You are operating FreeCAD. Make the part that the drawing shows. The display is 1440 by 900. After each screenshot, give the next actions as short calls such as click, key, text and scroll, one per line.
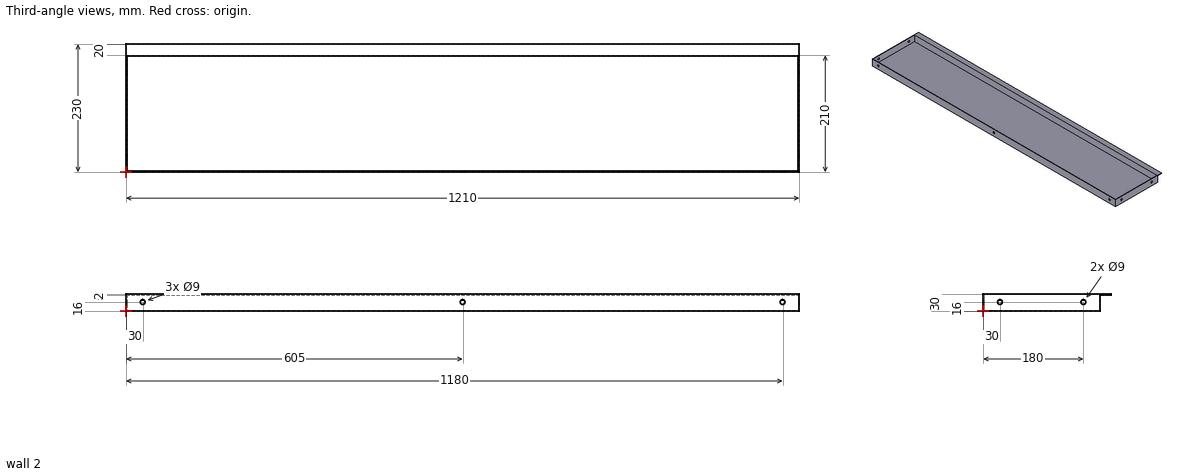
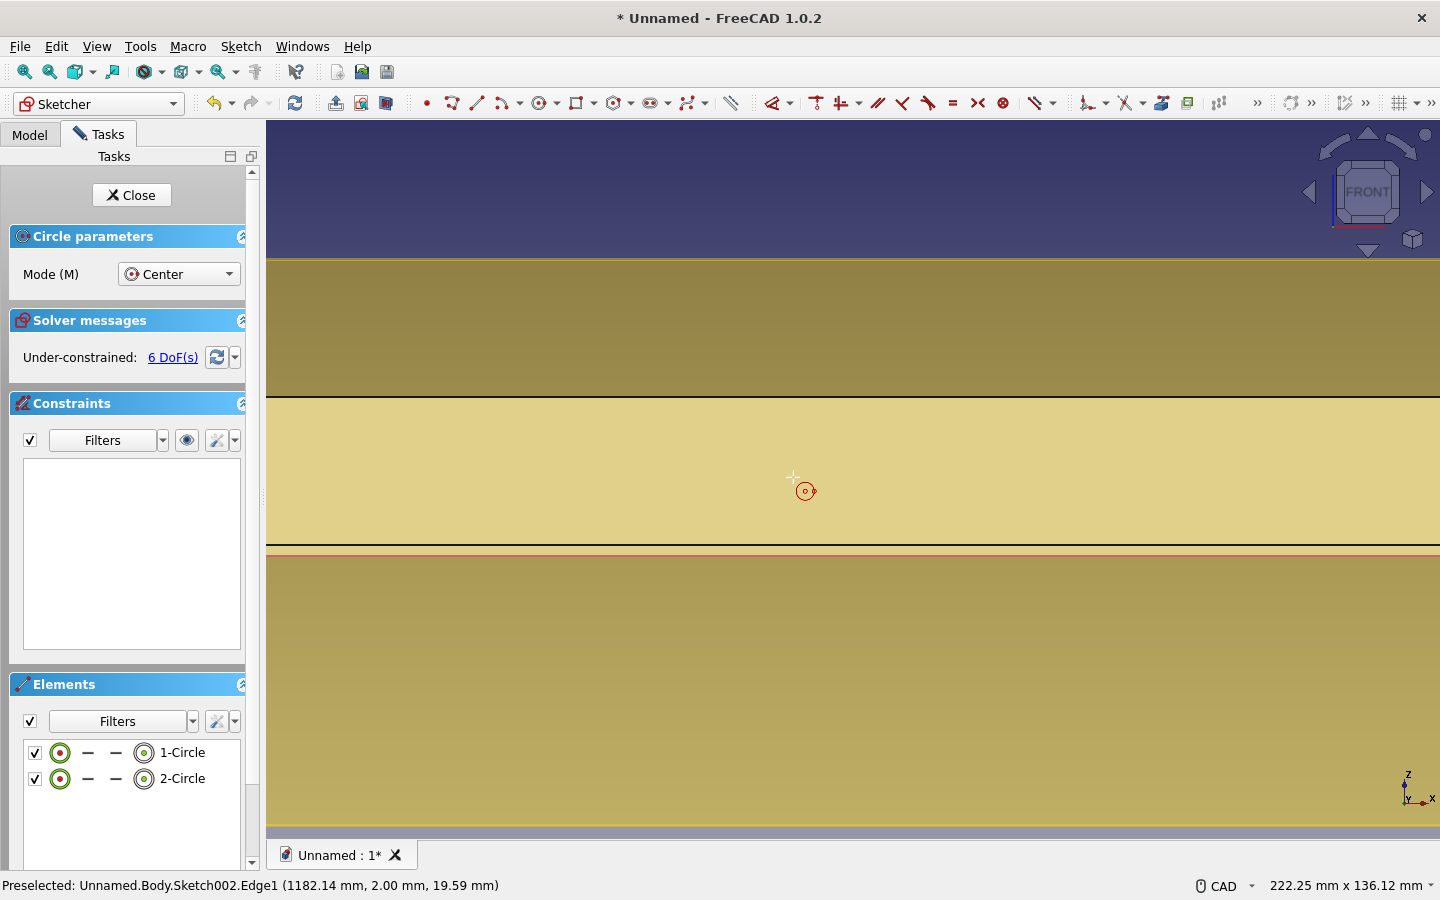
scroll(793, 477, down, 11)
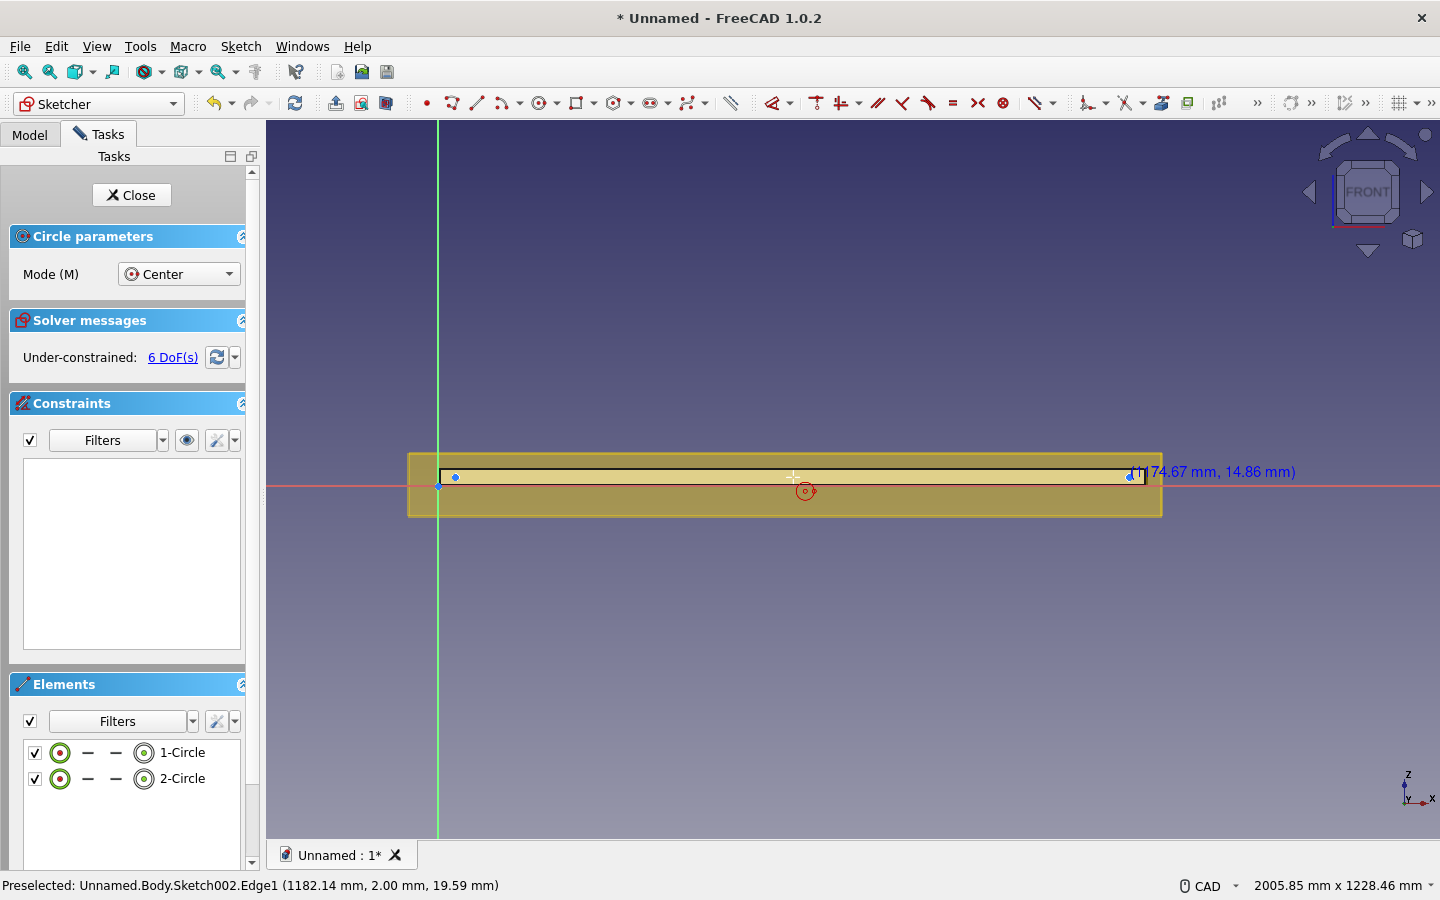
scroll(793, 477, up, 3)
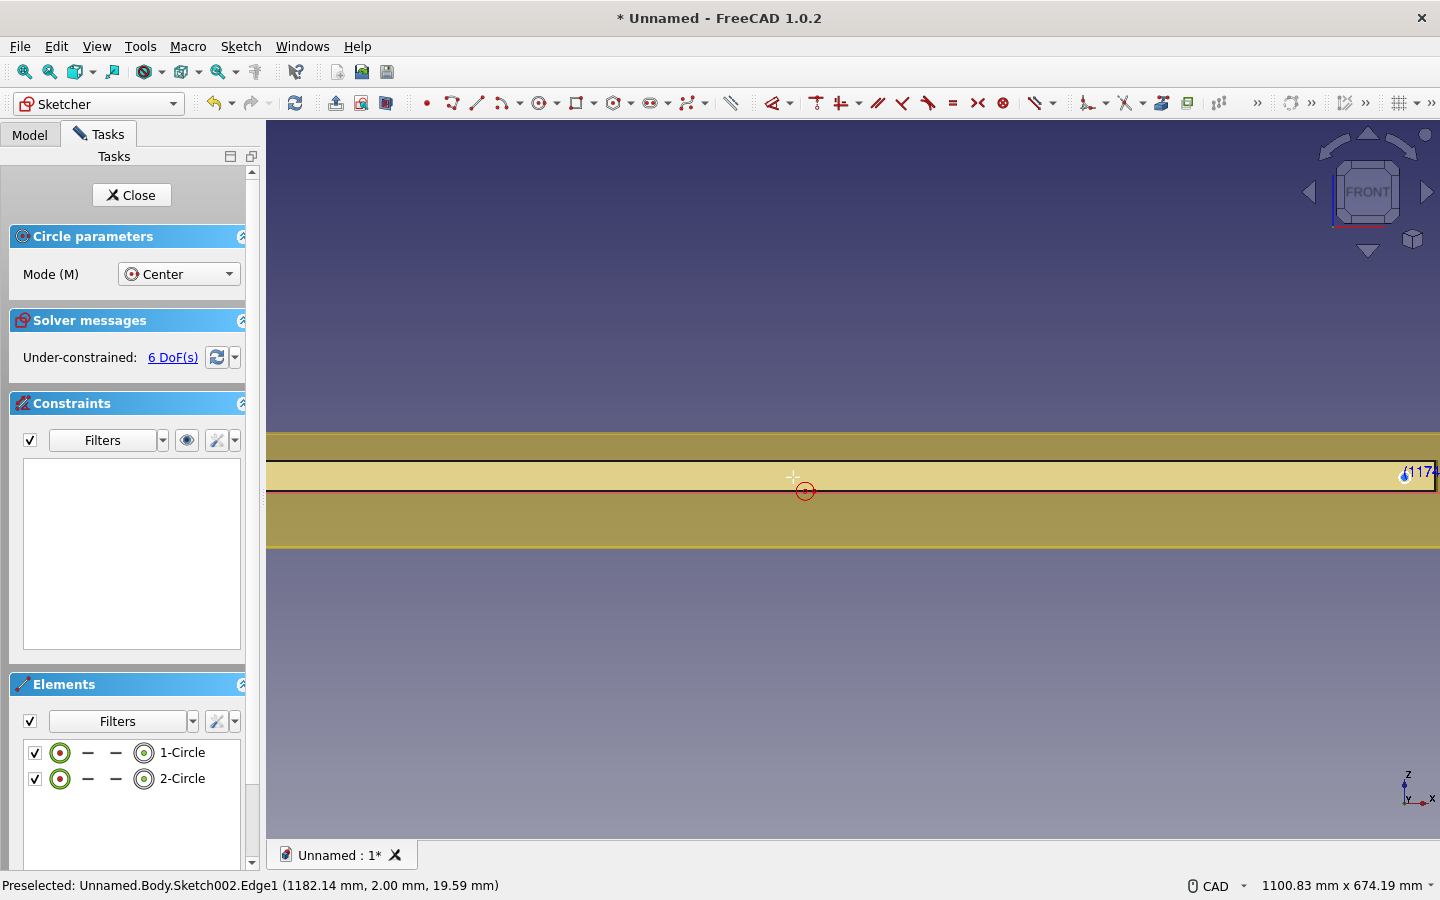
click(792, 476)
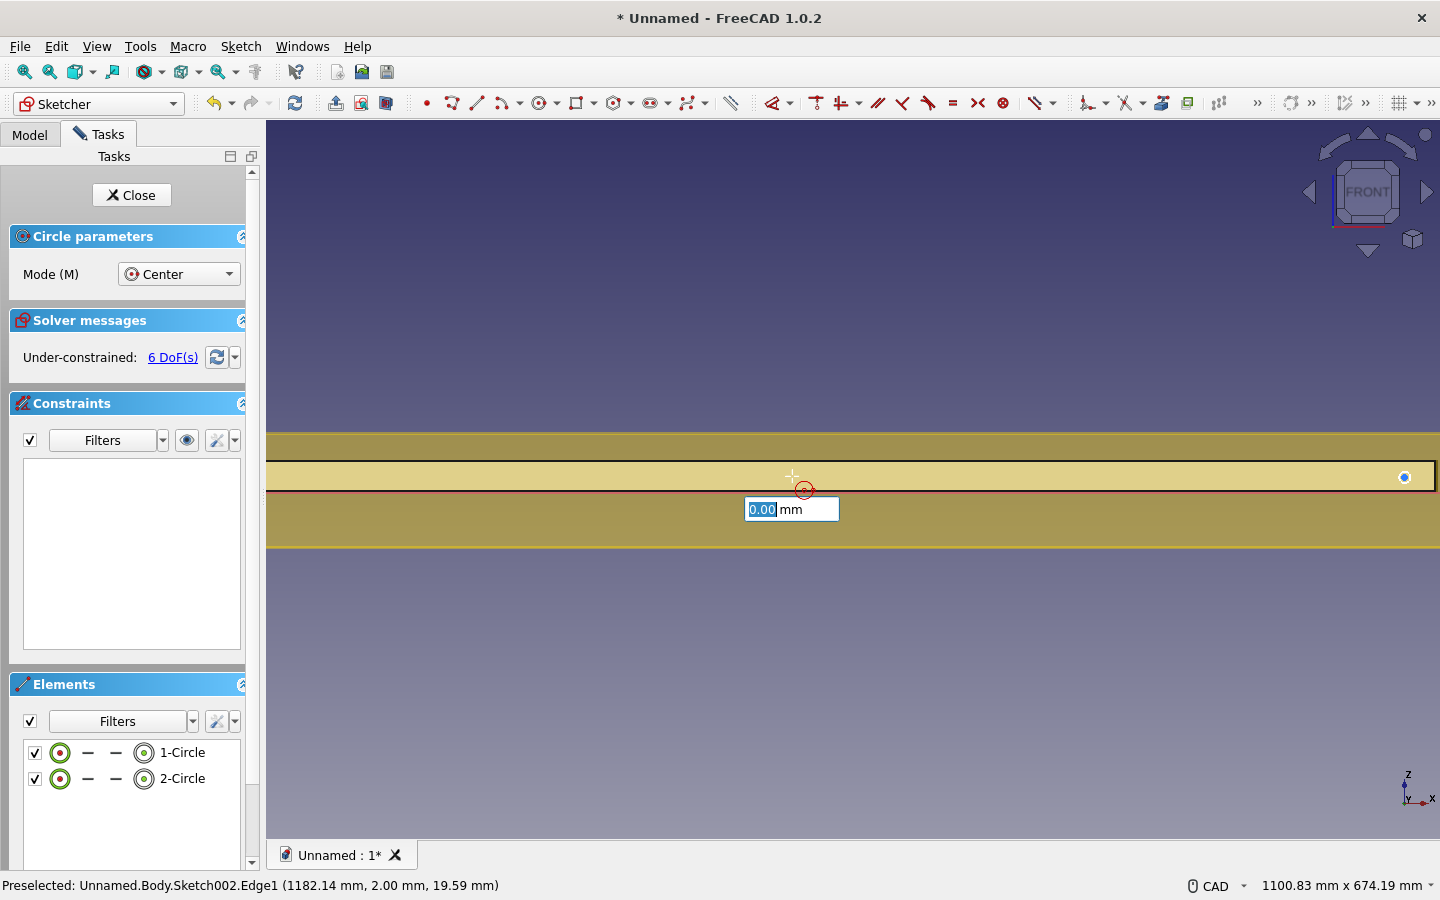
scroll(795, 473, up, 6)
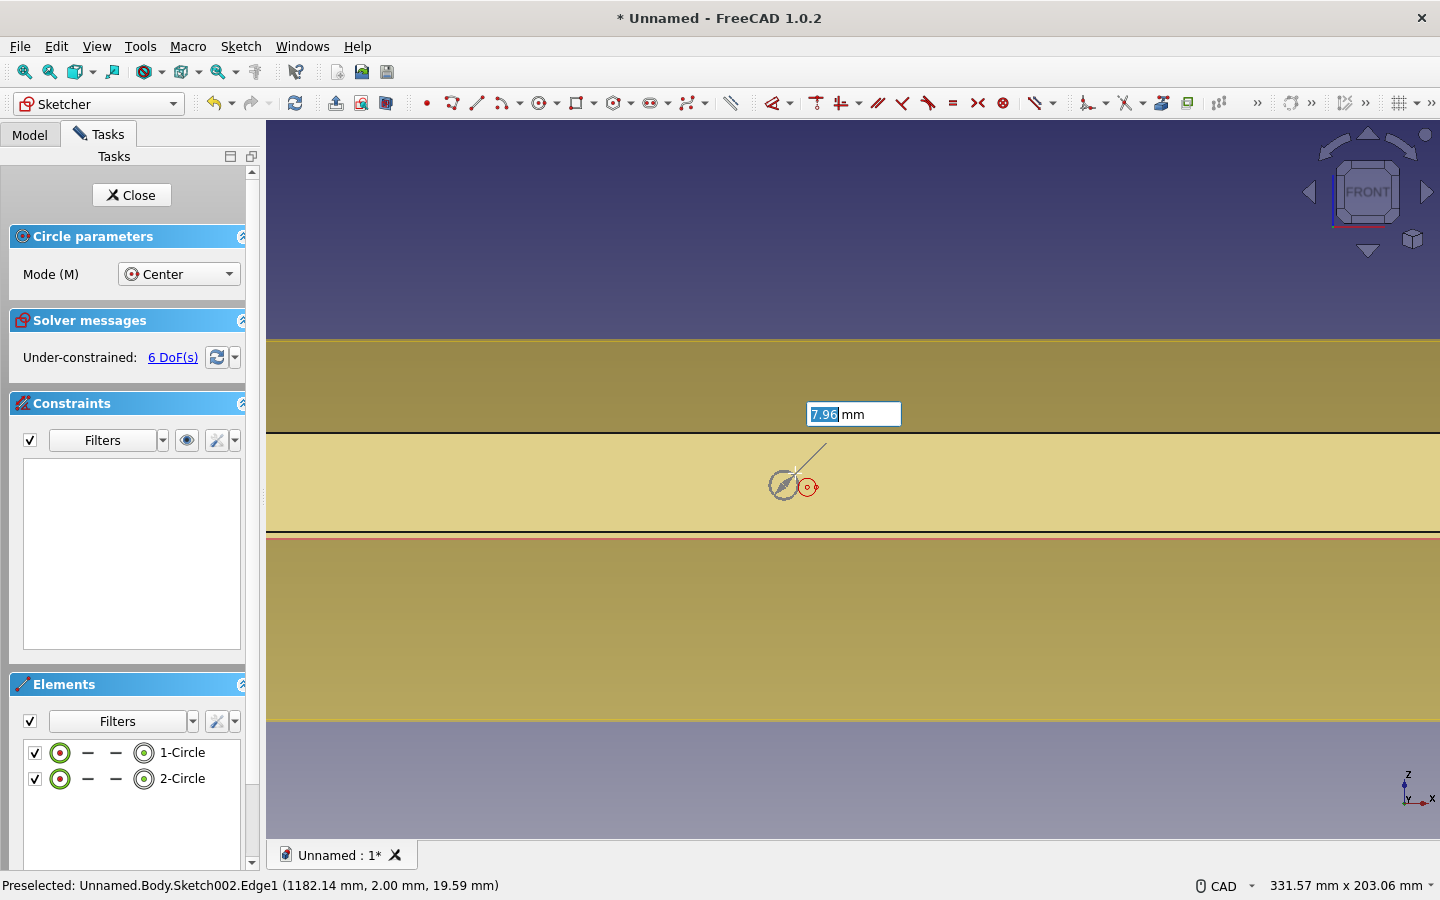
click(794, 471)
key(Escape)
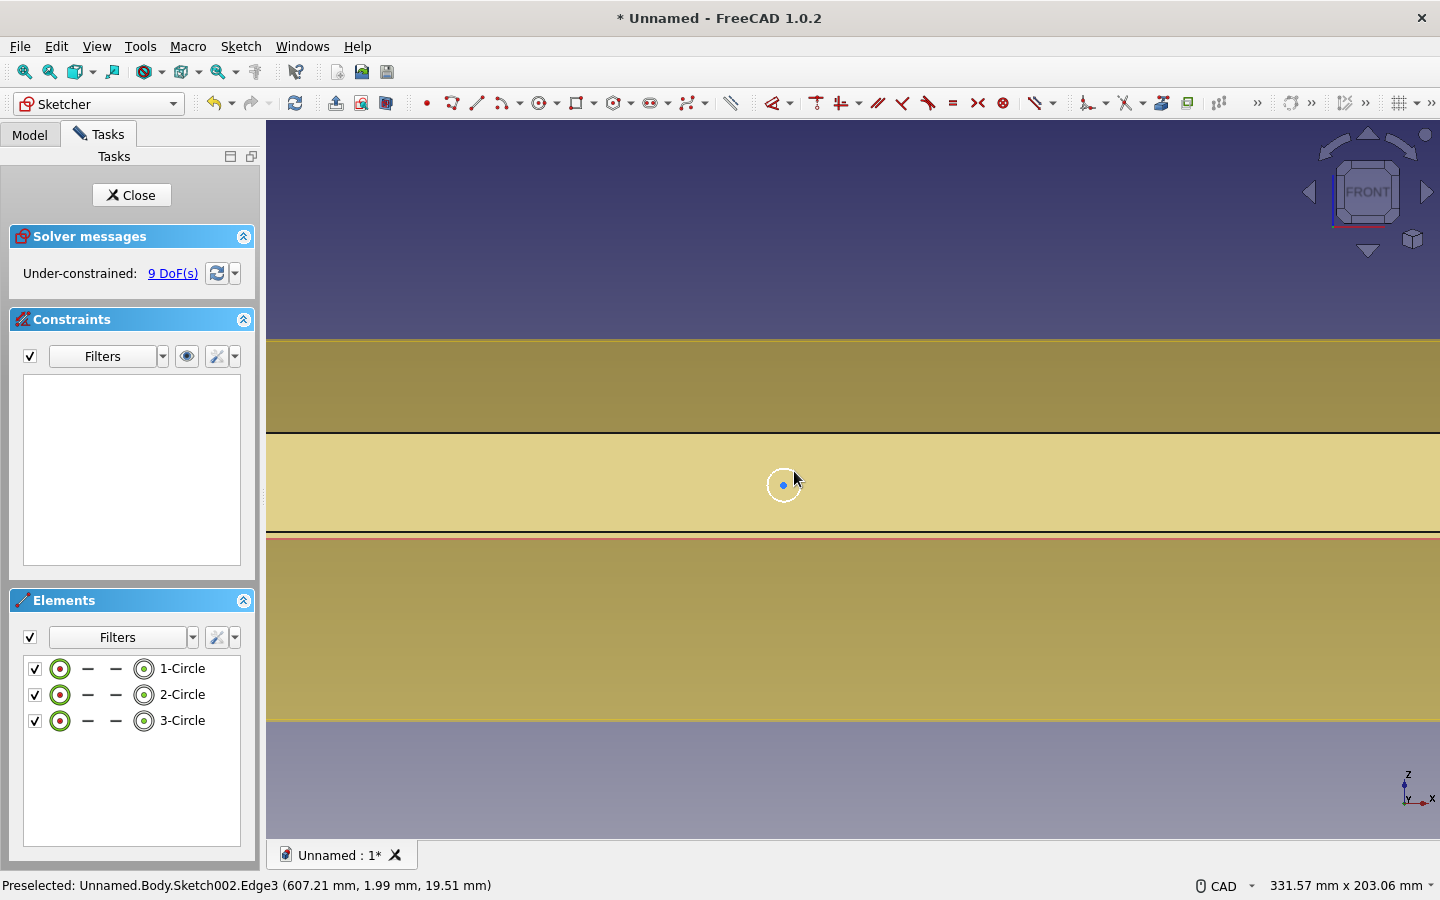
scroll(794, 475, down, 9)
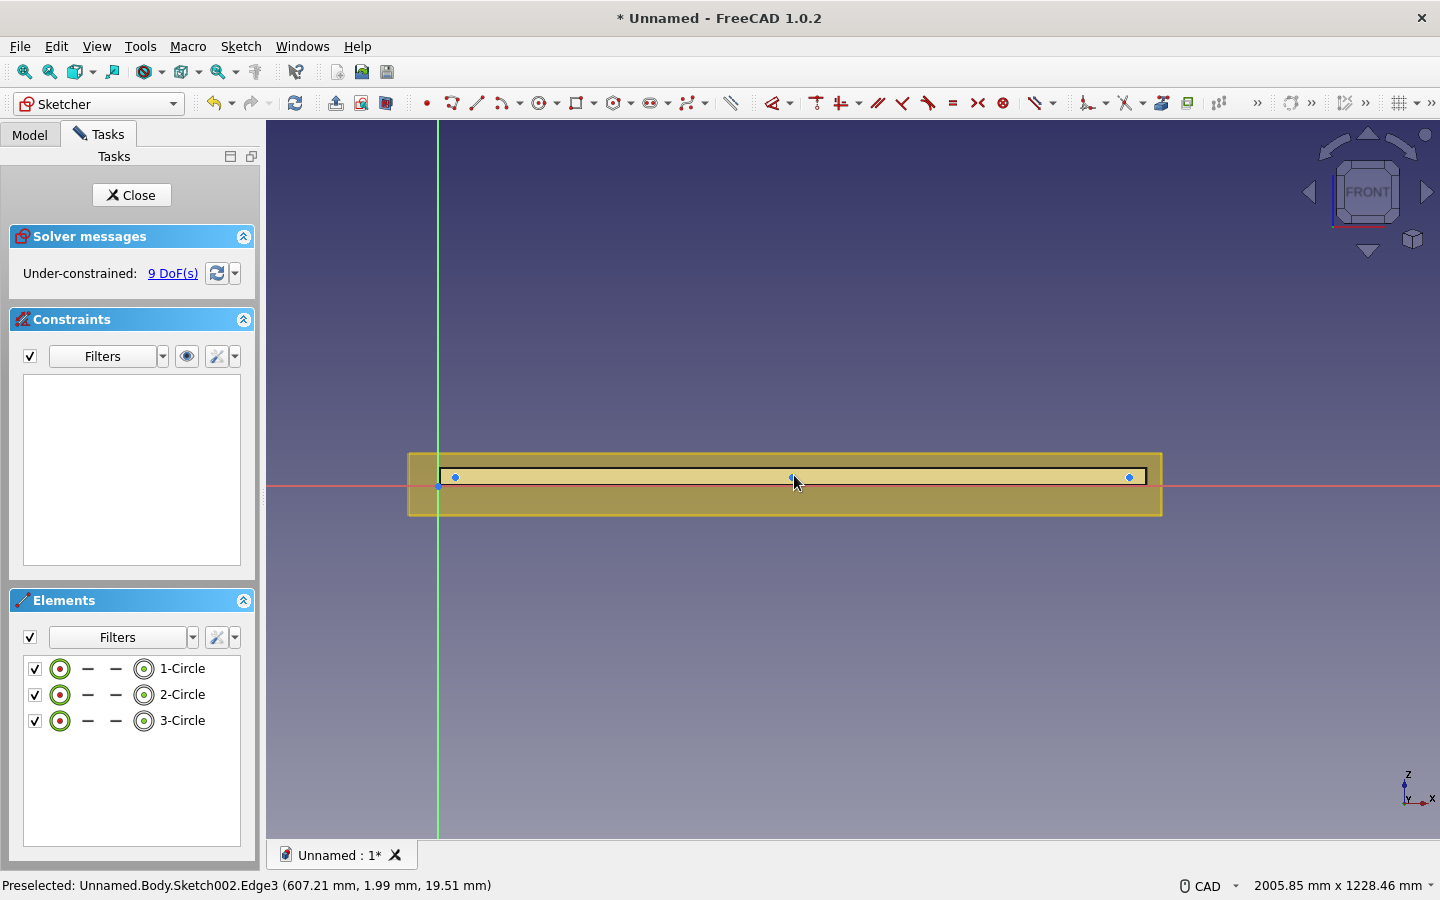
scroll(458, 475, up, 8)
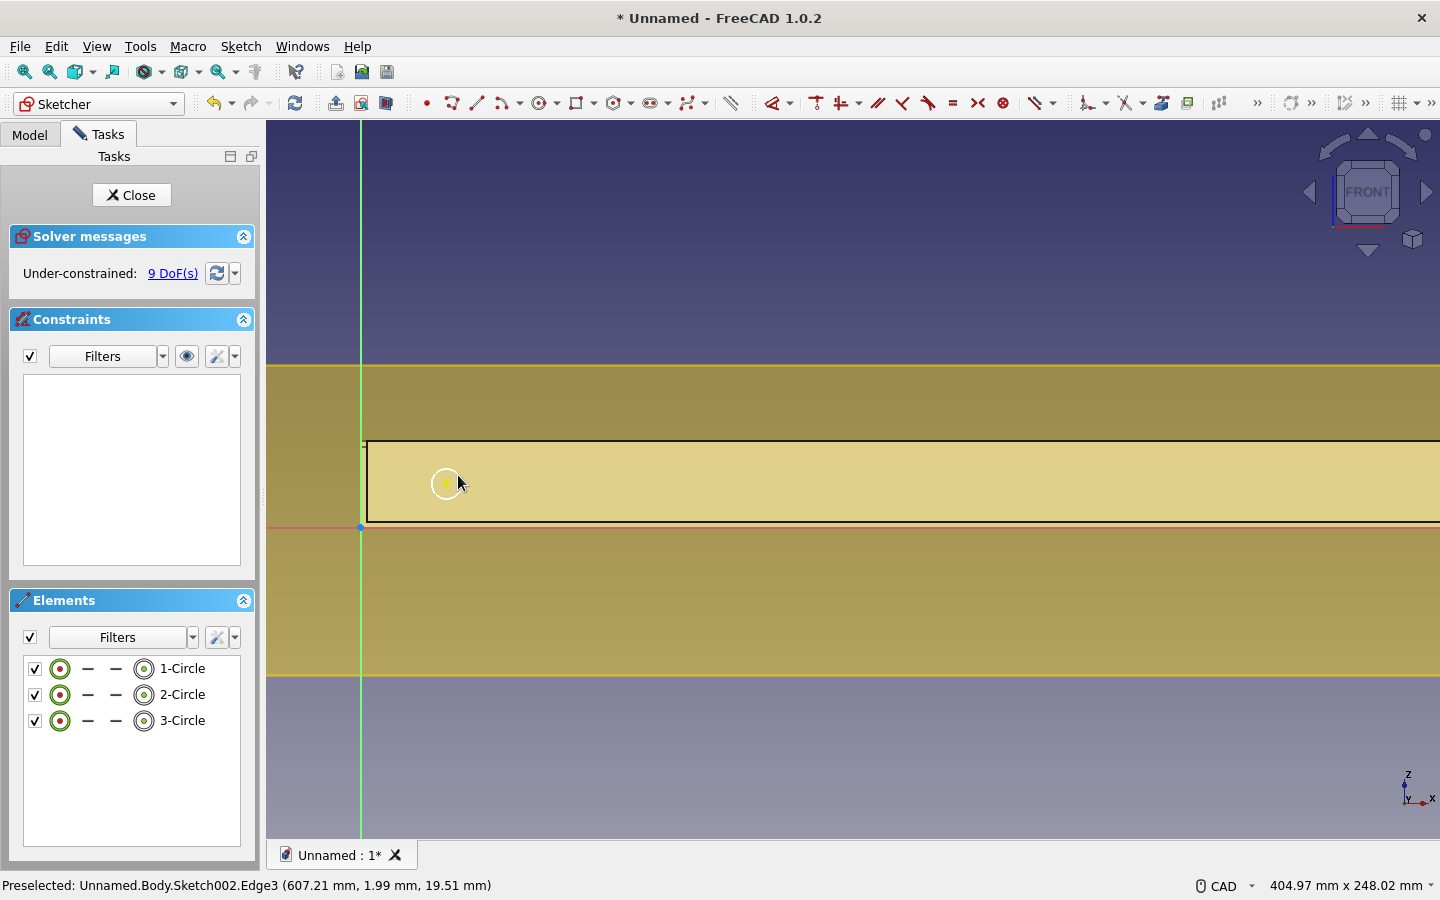
click(457, 473)